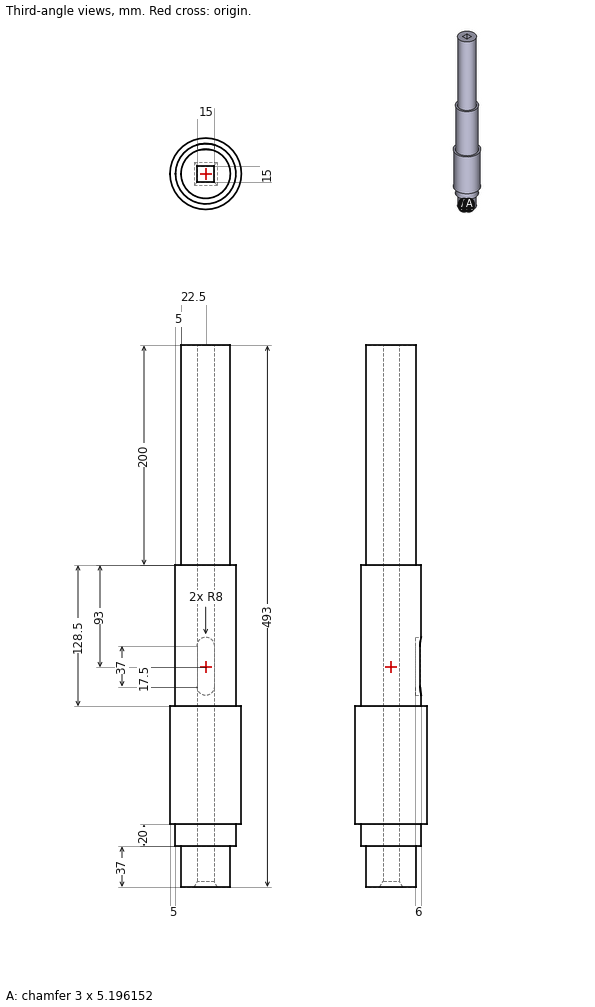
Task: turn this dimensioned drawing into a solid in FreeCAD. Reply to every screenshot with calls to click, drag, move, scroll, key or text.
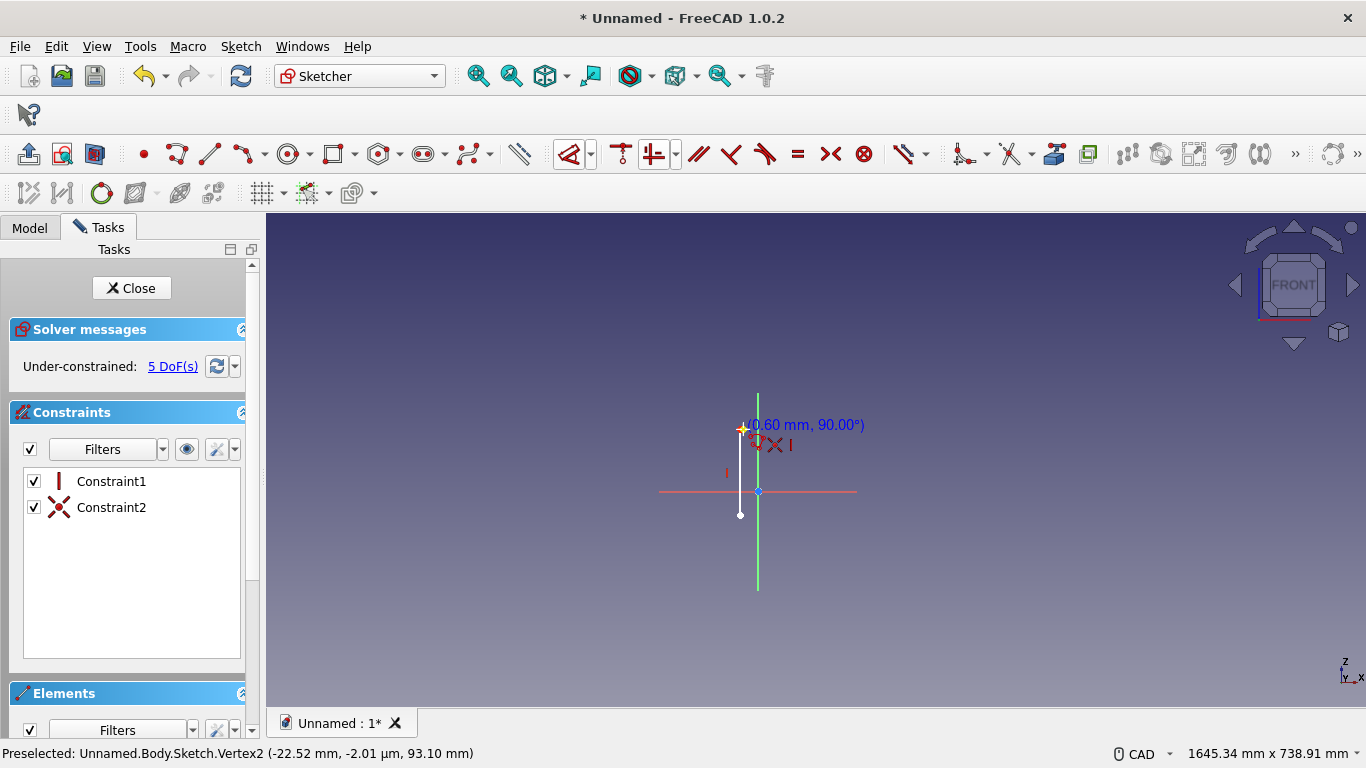
click(743, 296)
click(758, 296)
click(749, 625)
click(743, 625)
click(743, 601)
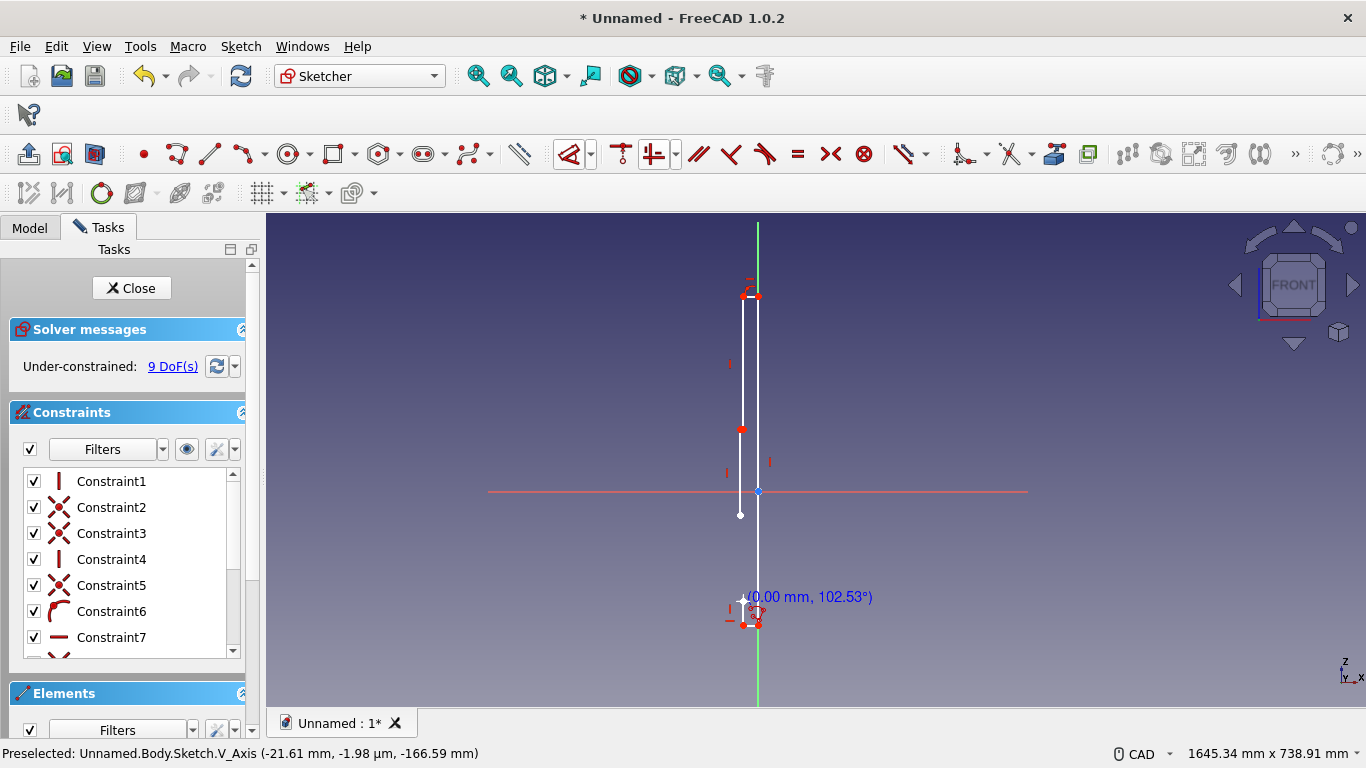
scroll(740, 601, up, 8)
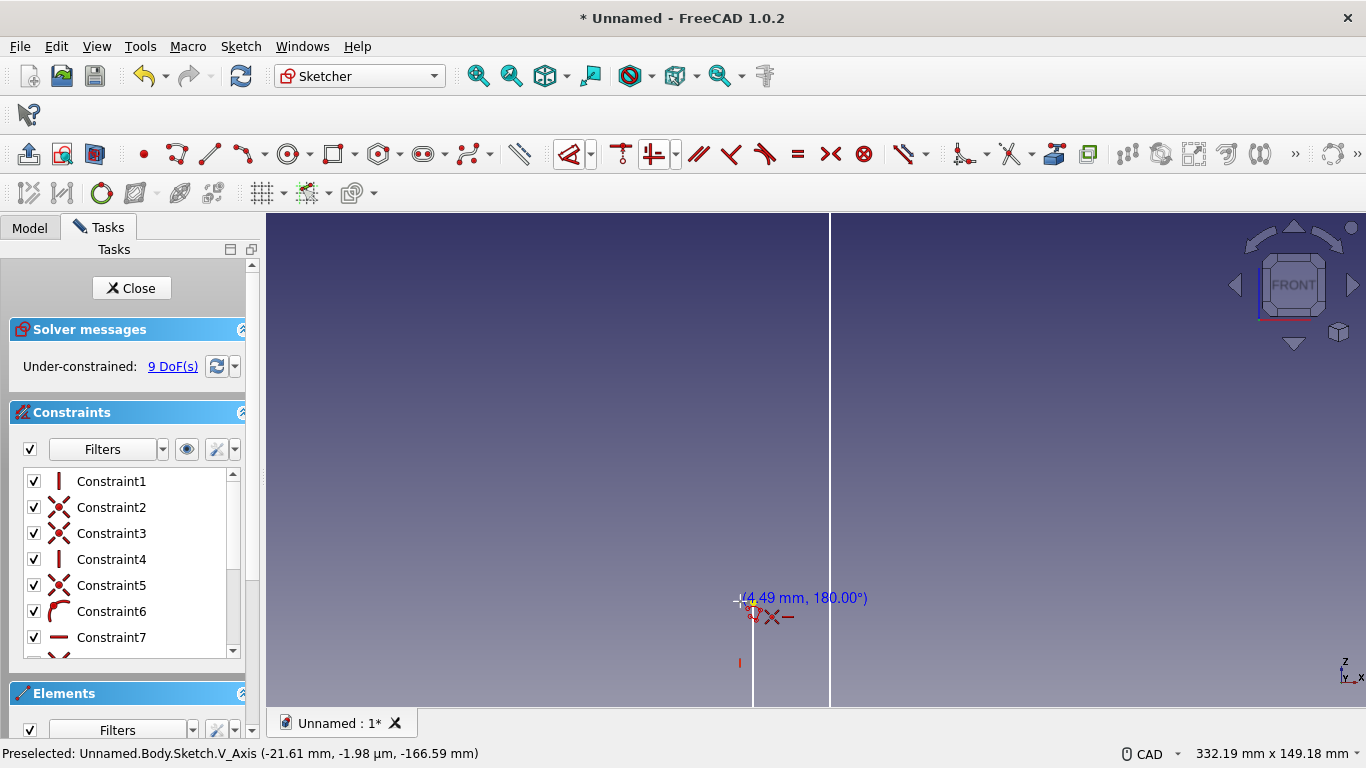
click(739, 598)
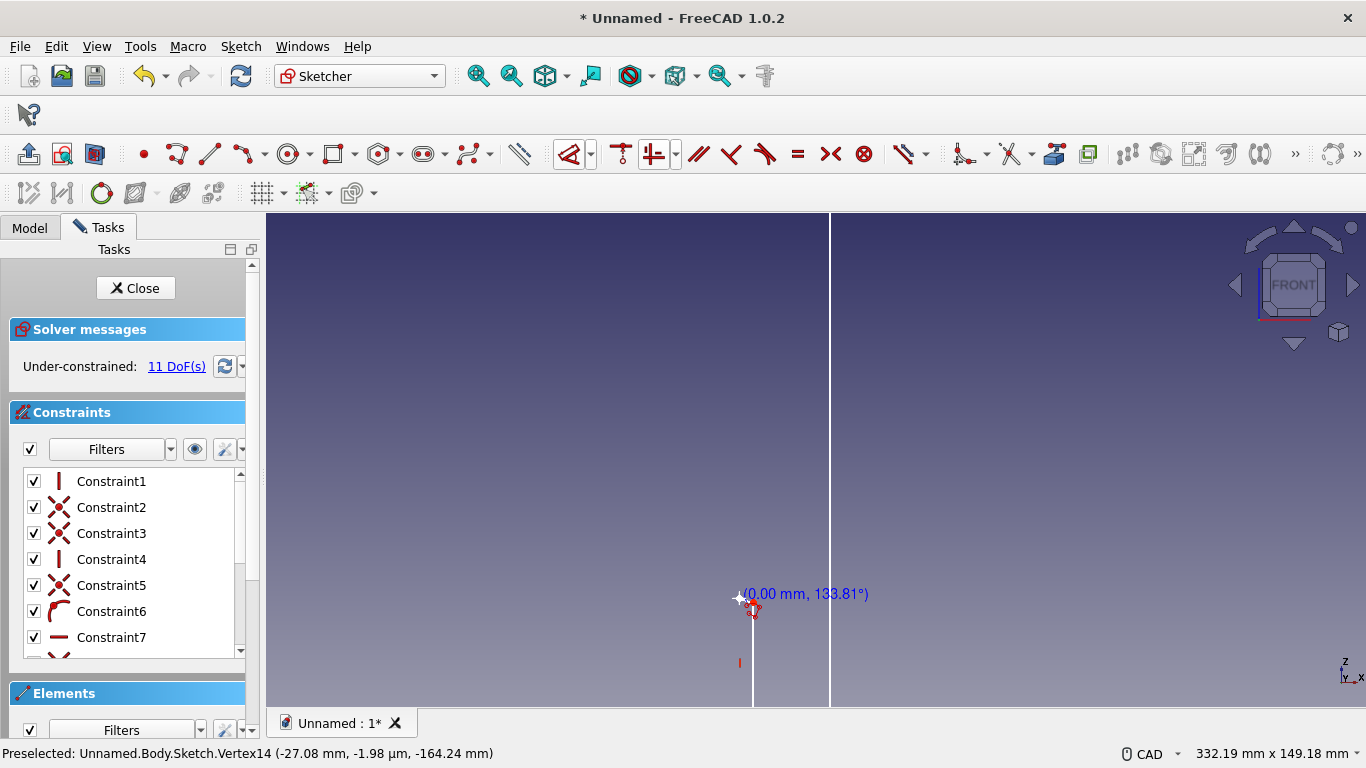
scroll(740, 601, down, 8)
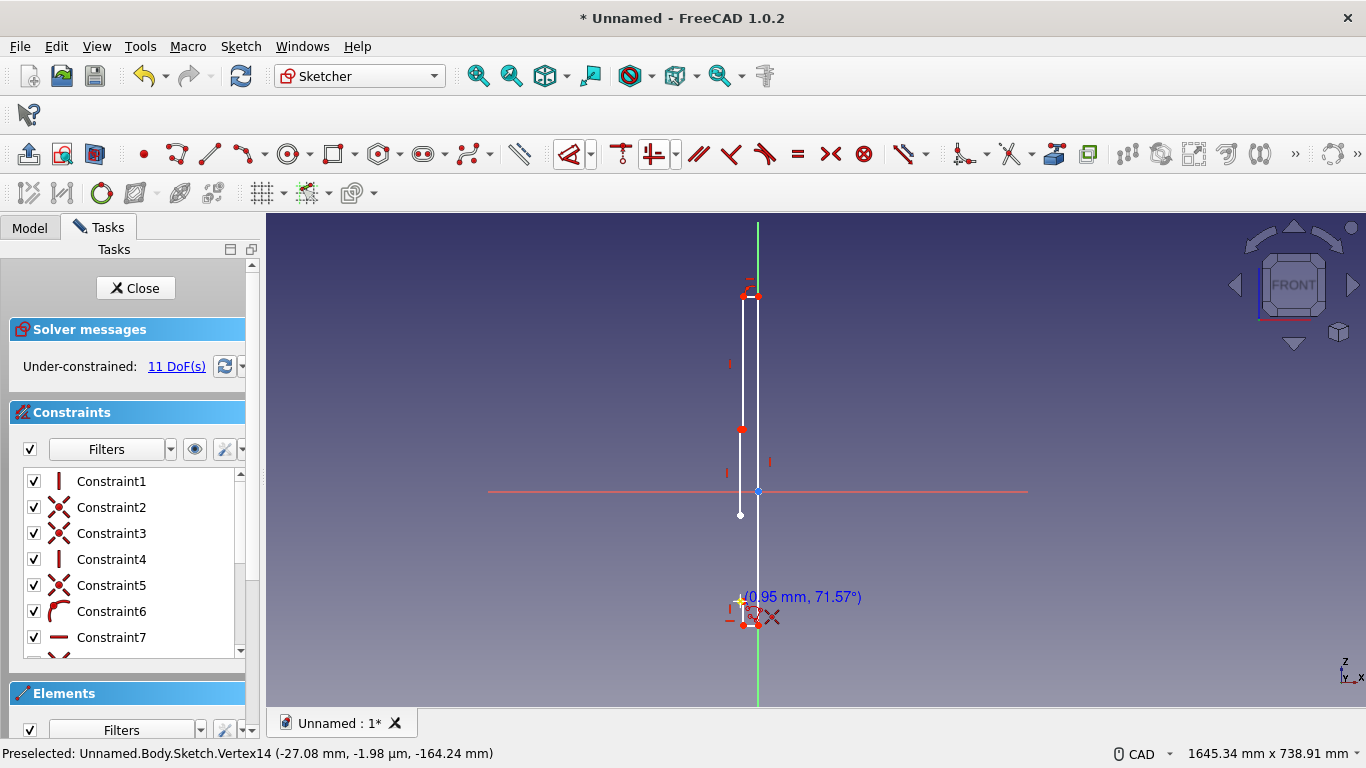
click(740, 587)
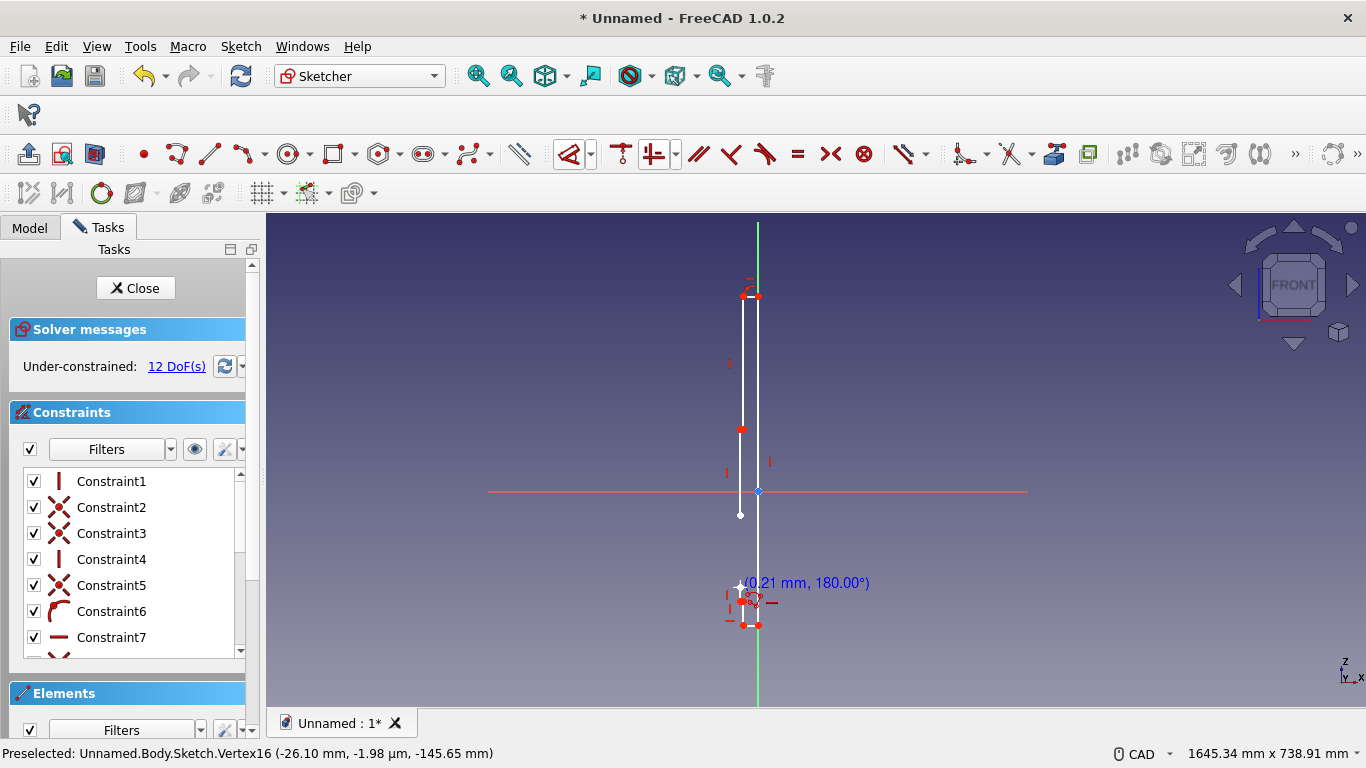
scroll(737, 587, up, 8)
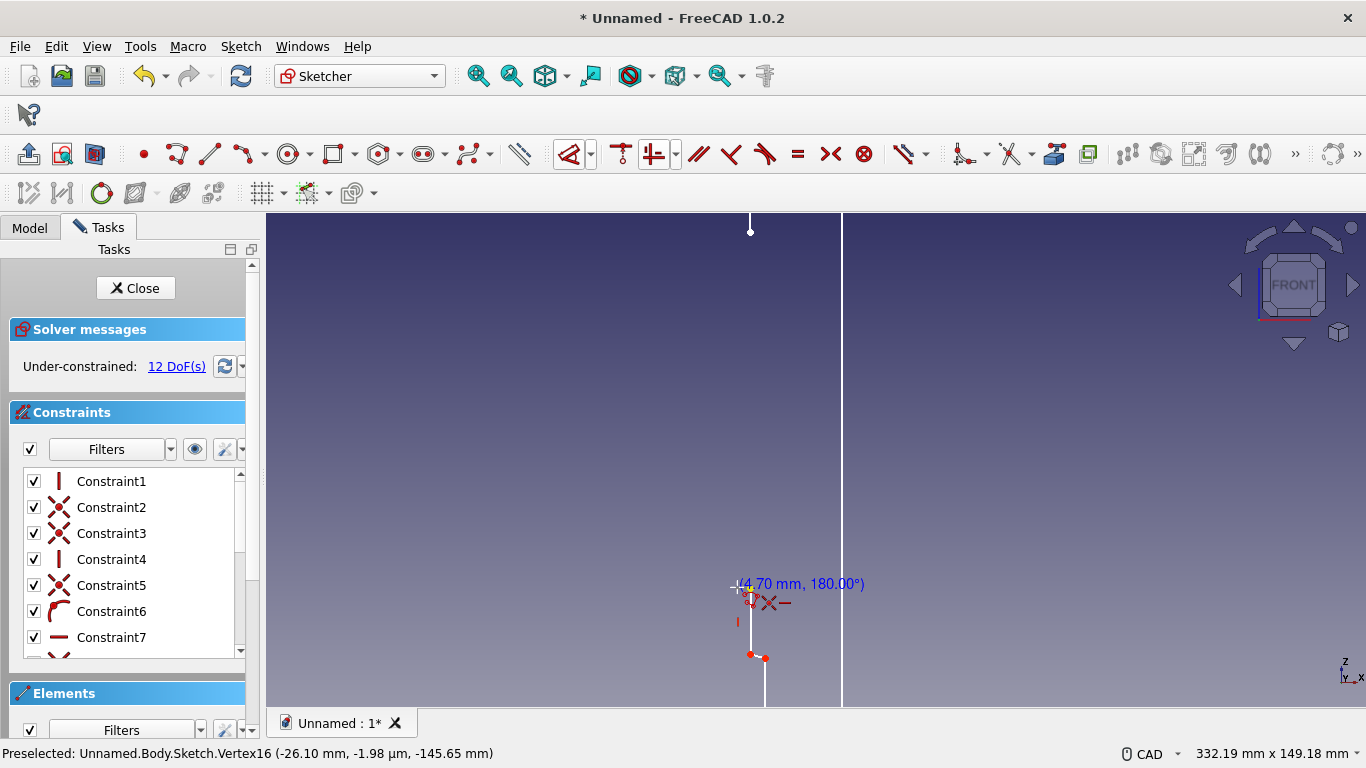
click(734, 584)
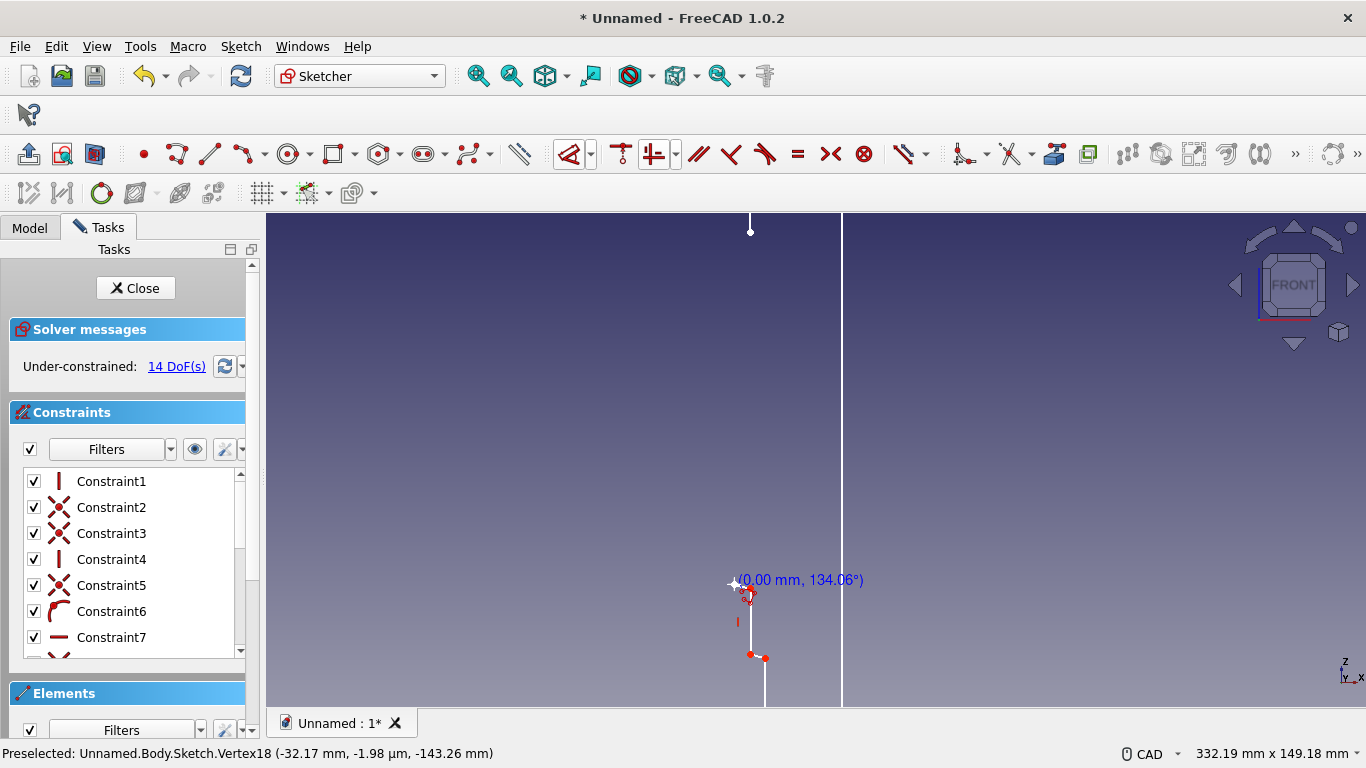
scroll(737, 587, down, 8)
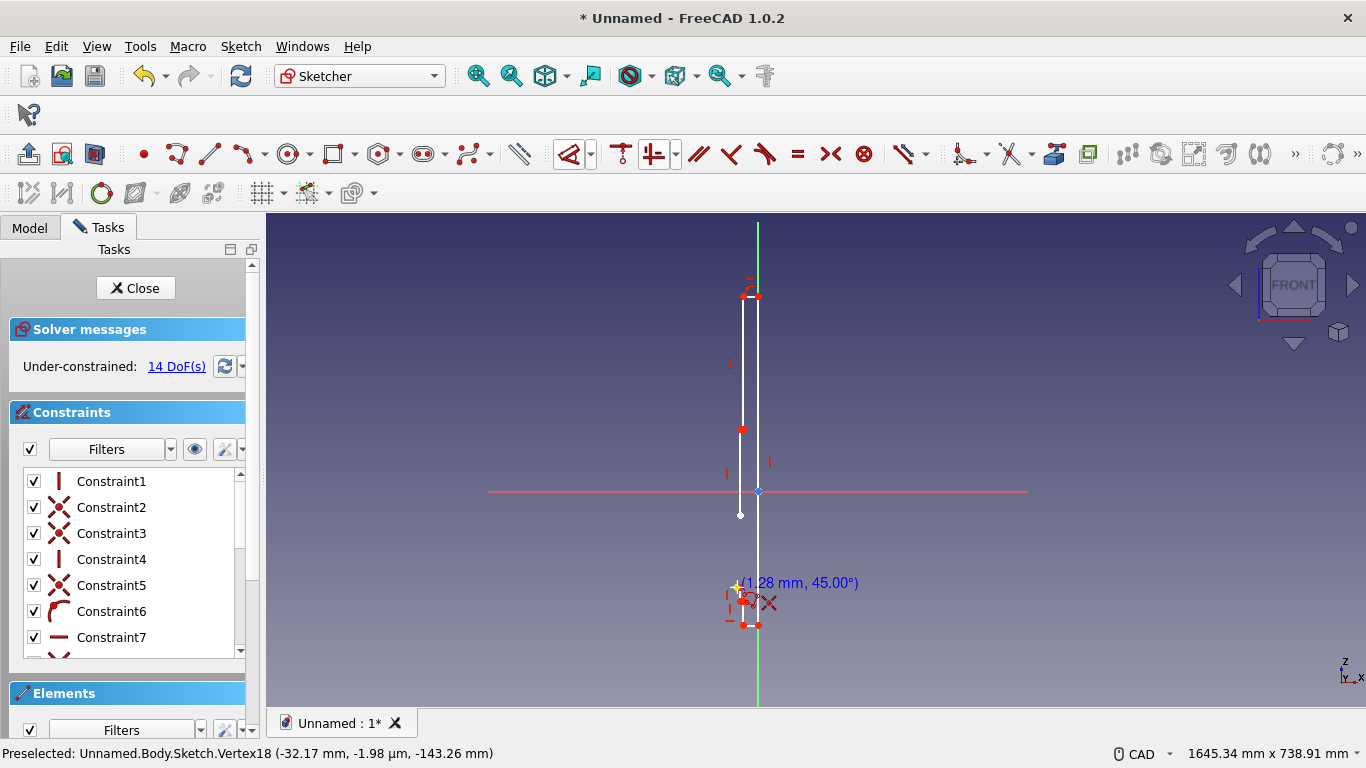
scroll(737, 515, up, 8)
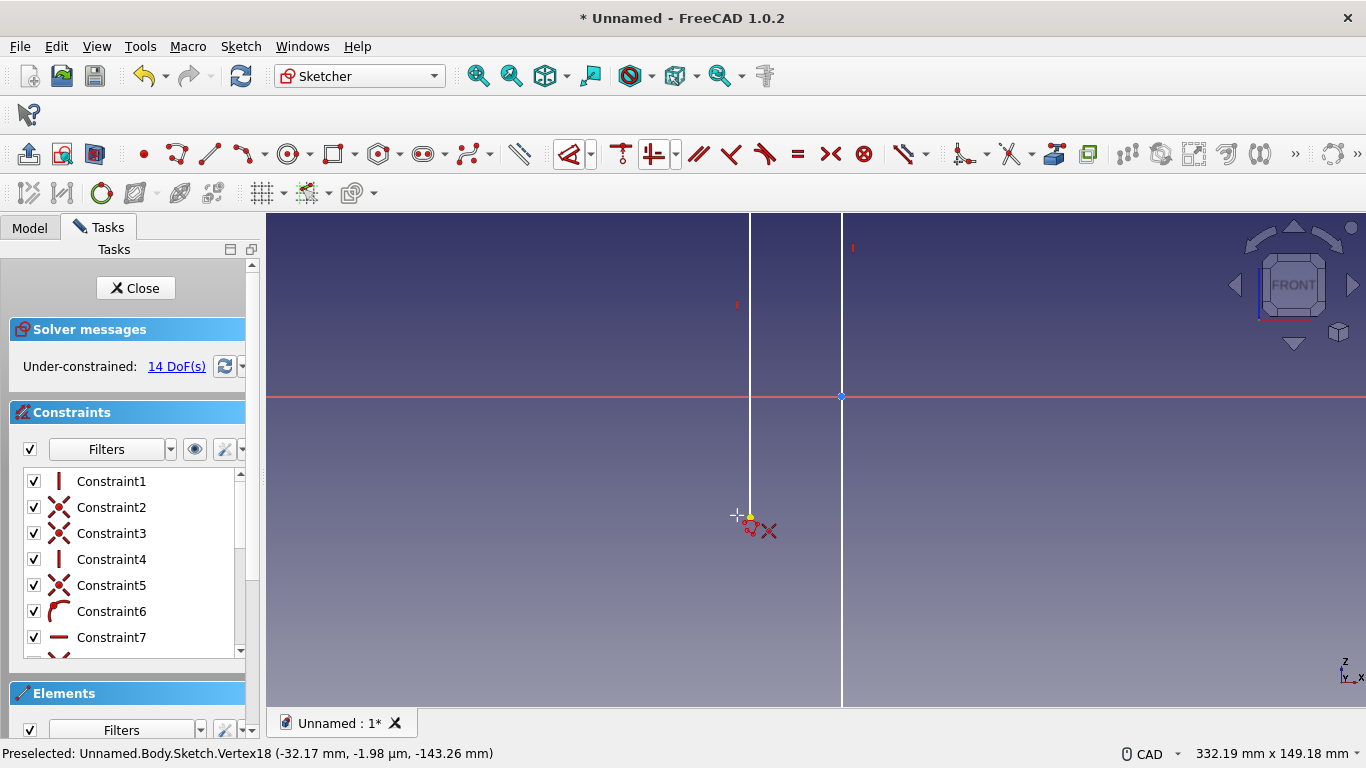
click(734, 514)
click(750, 518)
key(Escape)
key(Escape)